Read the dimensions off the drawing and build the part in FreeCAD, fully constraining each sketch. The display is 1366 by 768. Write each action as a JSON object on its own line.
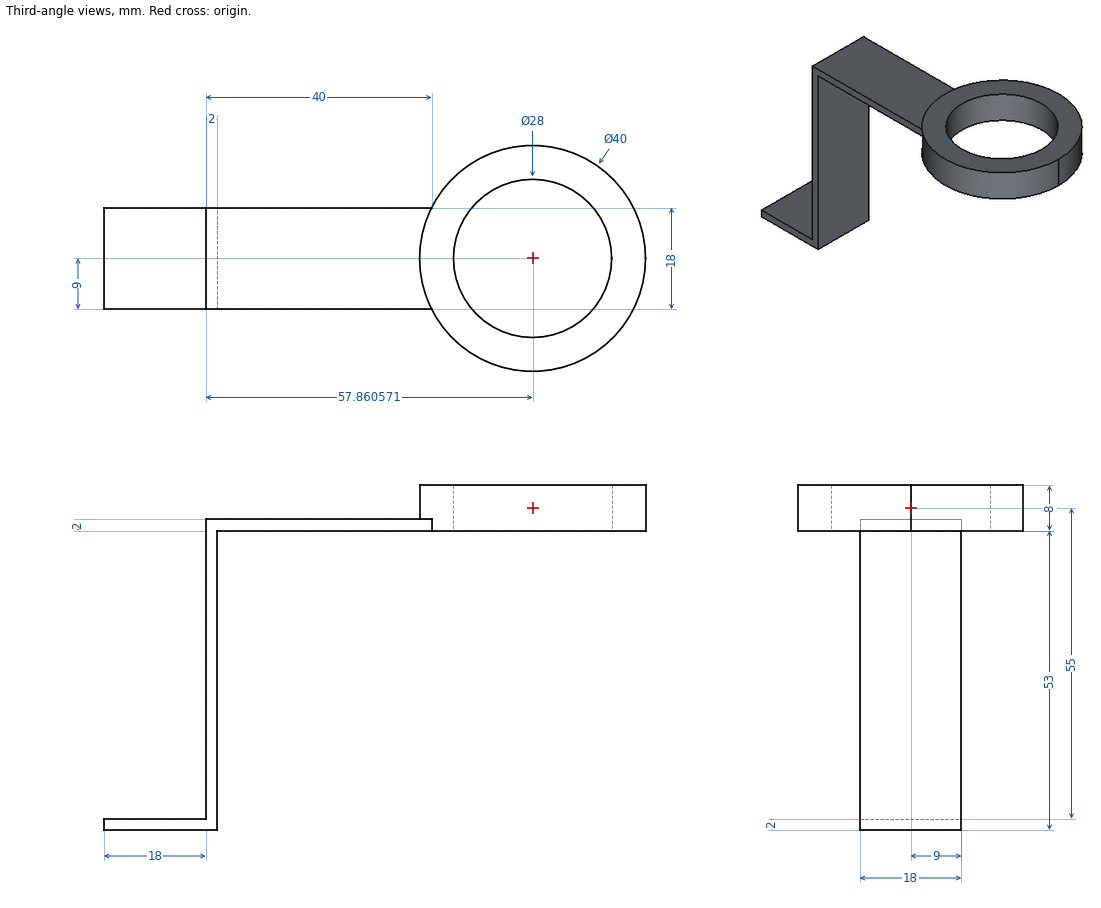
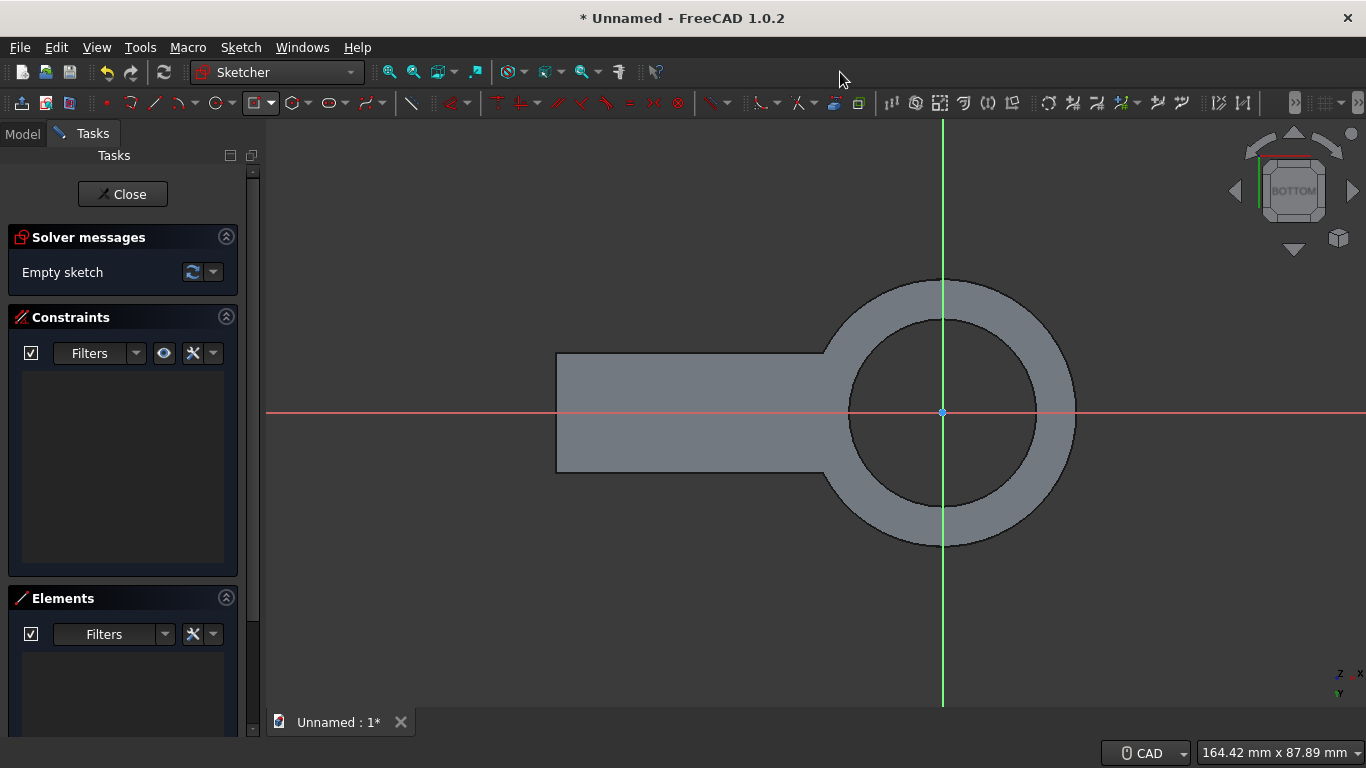
{"action": "scroll", "coordinate": [482, 413], "scroll_direction": "up", "scroll_amount": 6}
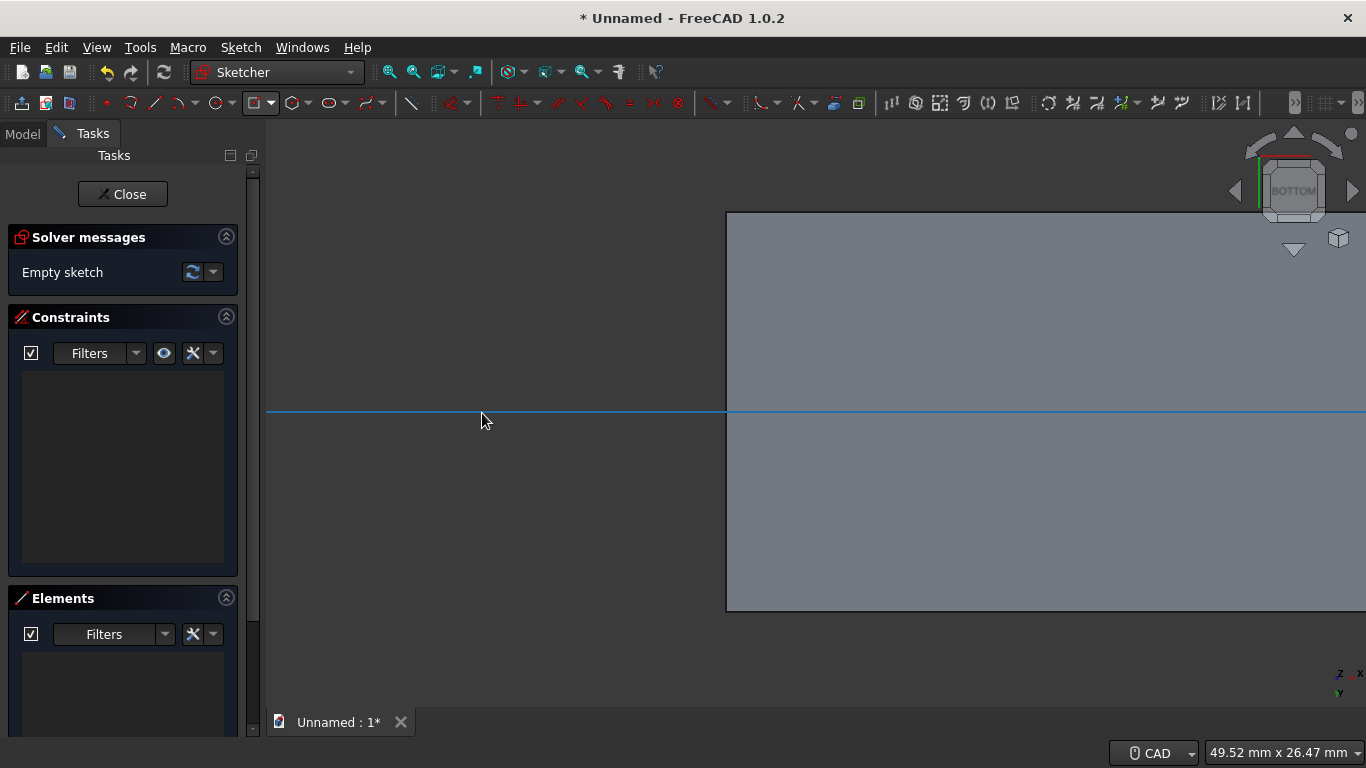
{"action": "left_click", "coordinate": [274, 104]}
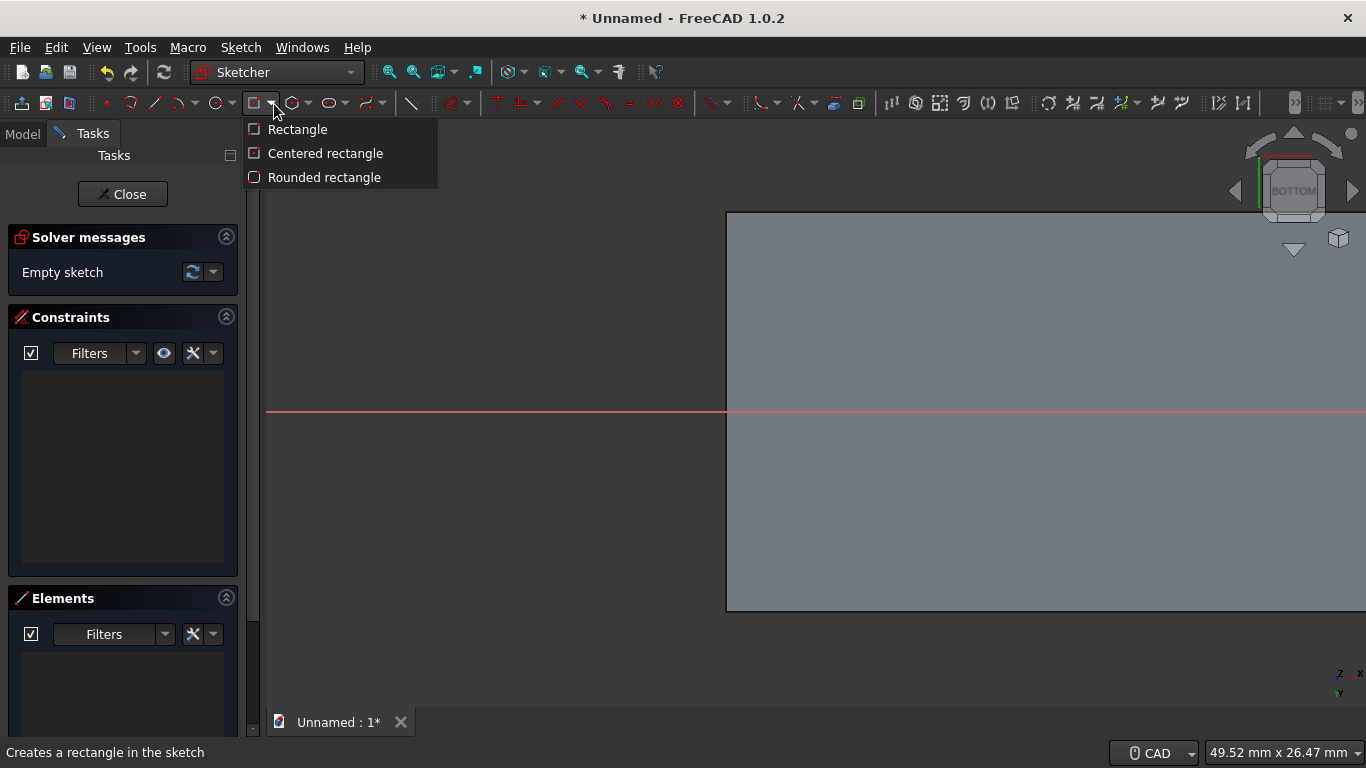
{"action": "left_click", "coordinate": [340, 129]}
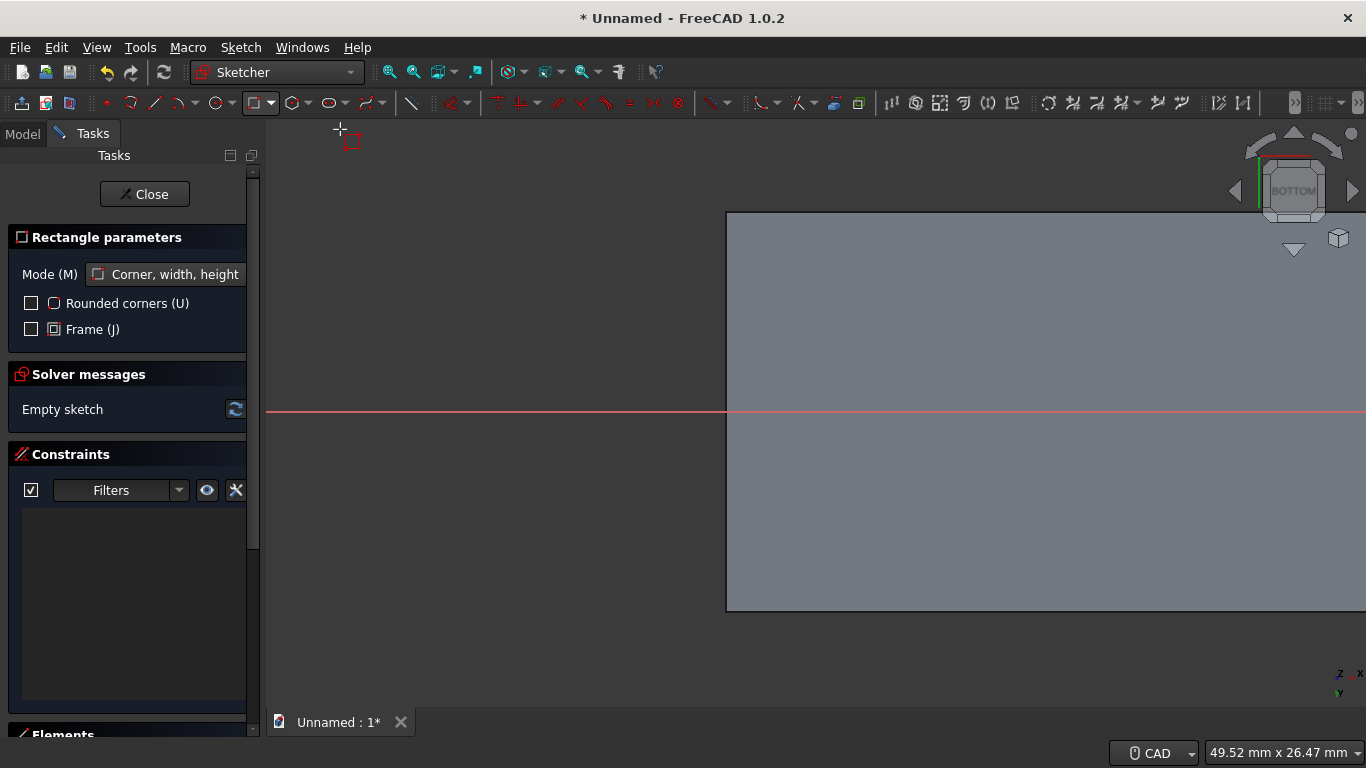
{"action": "left_click", "coordinate": [726, 212]}
{"action": "mouse_move", "coordinate": [770, 612]}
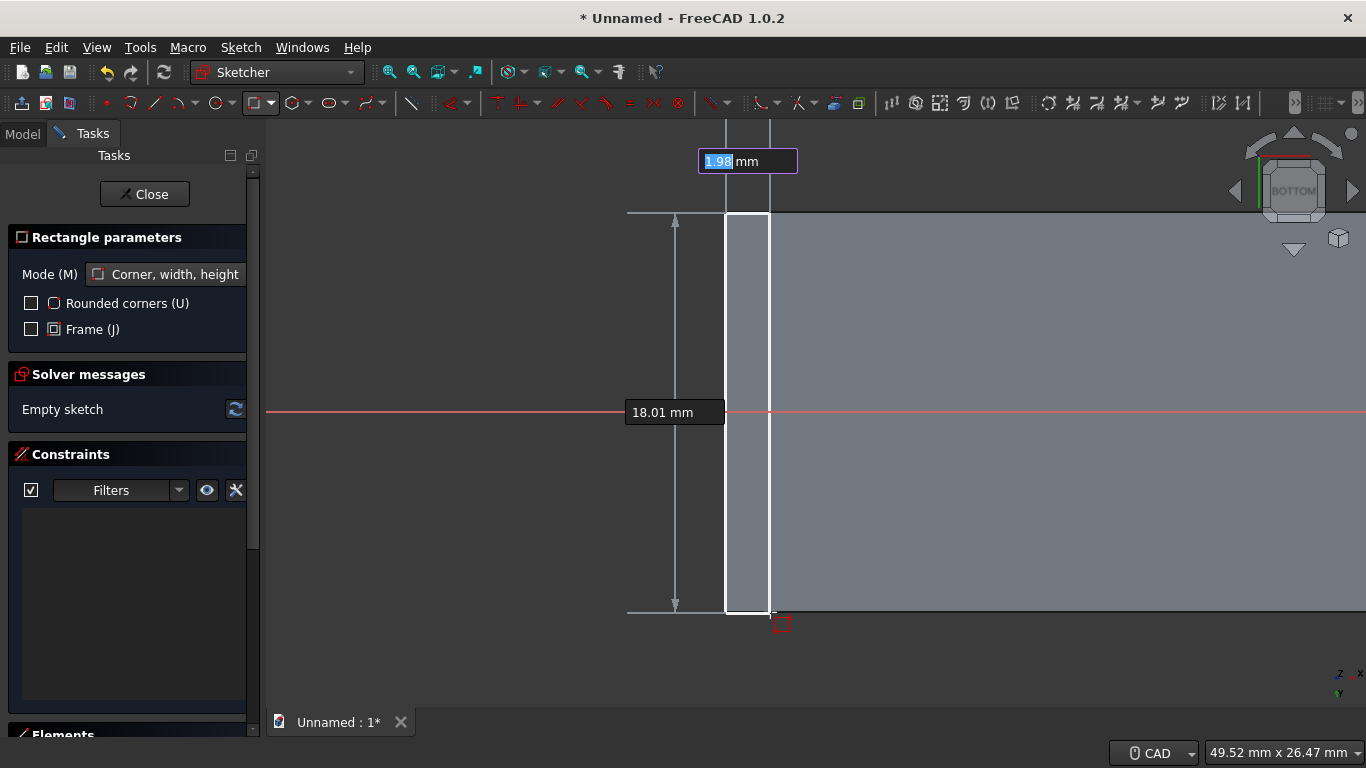
{"action": "type", "text": "2"}
{"action": "key", "text": "Tab"}
{"action": "type", "text": "18"}
{"action": "key", "text": "Return"}
{"action": "key", "text": "Escape"}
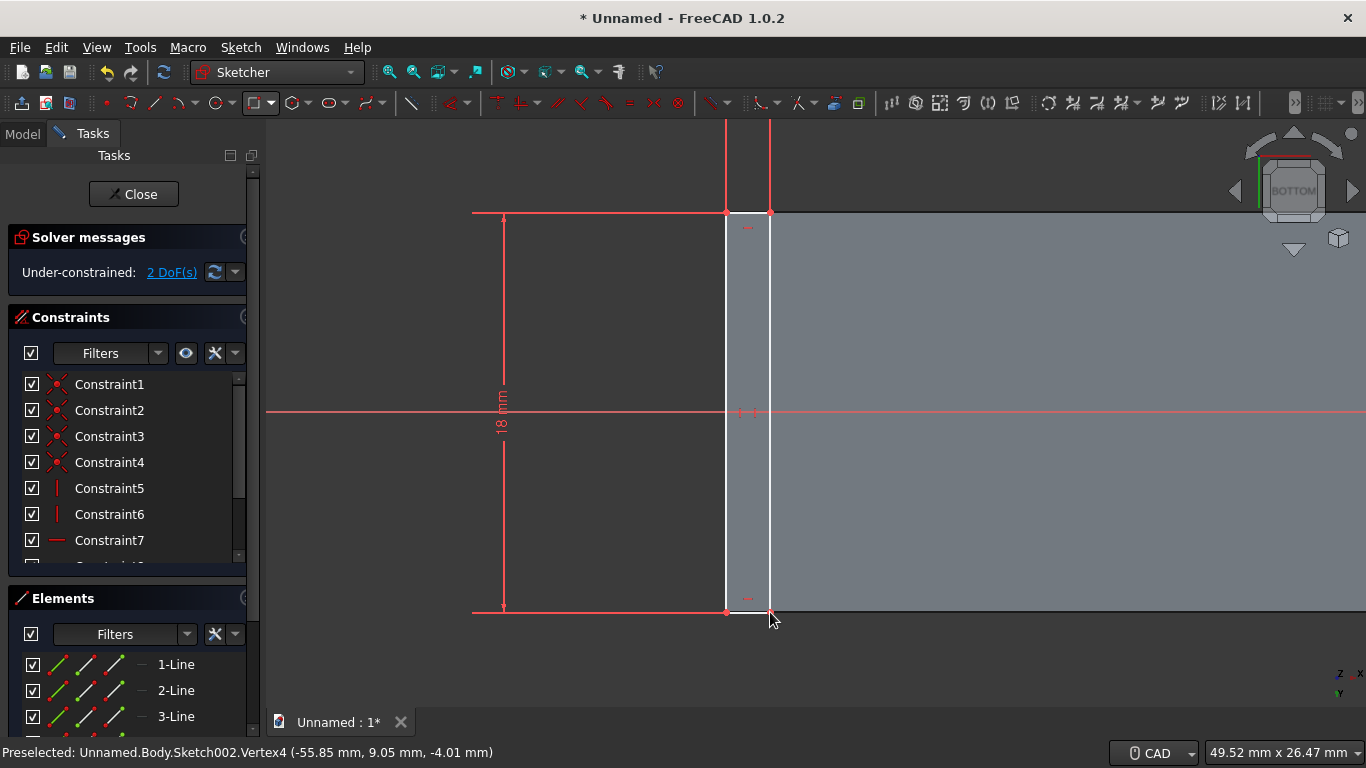
{"action": "left_click", "coordinate": [450, 104]}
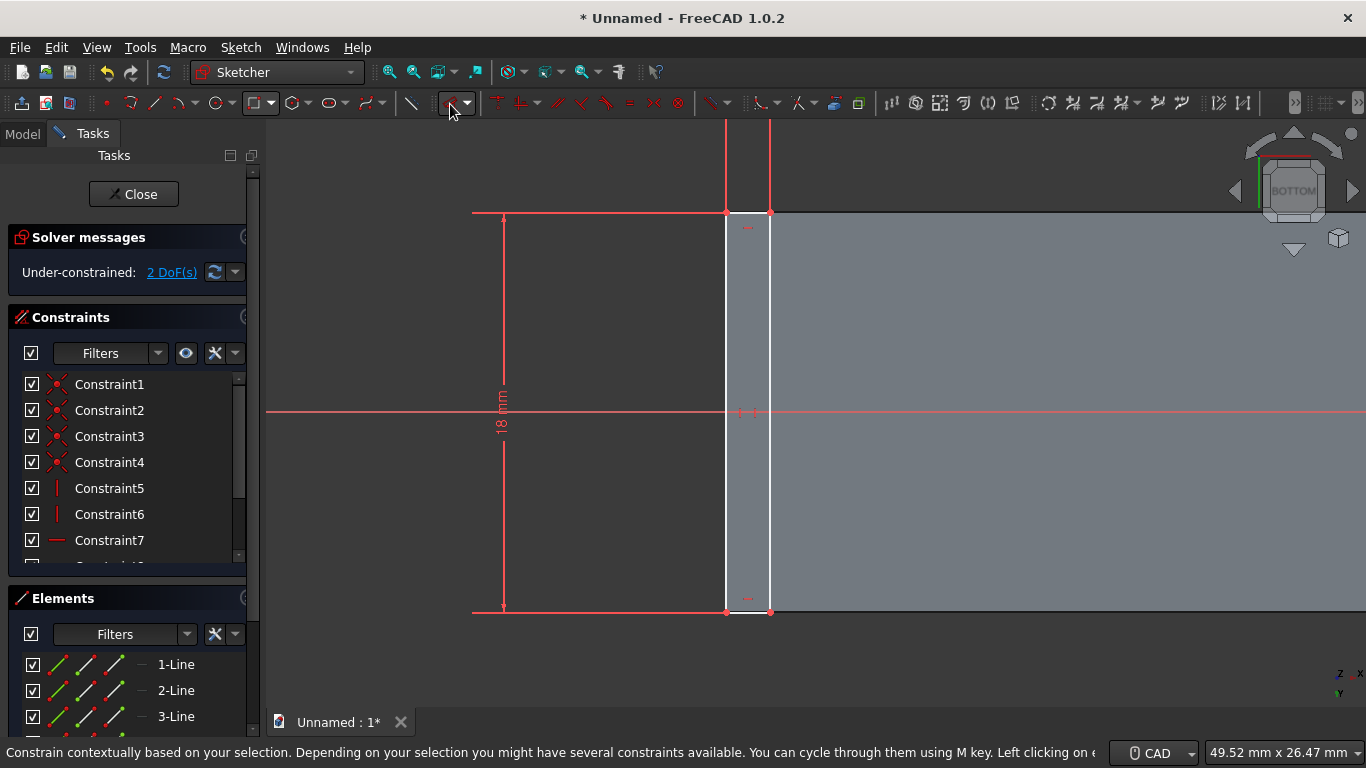
{"action": "left_click", "coordinate": [726, 213]}
{"action": "left_click", "coordinate": [692, 312]}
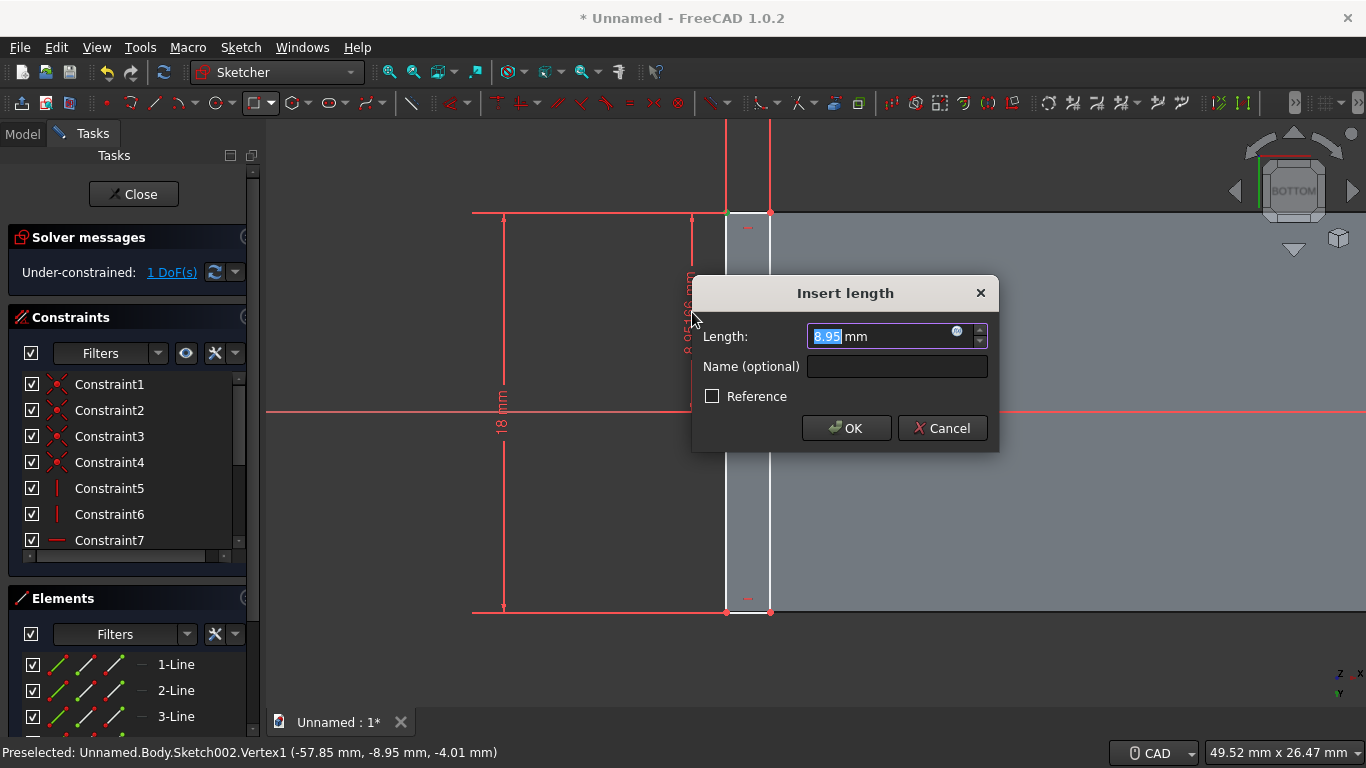
{"action": "type", "text": "9"}
{"action": "key", "text": "Return"}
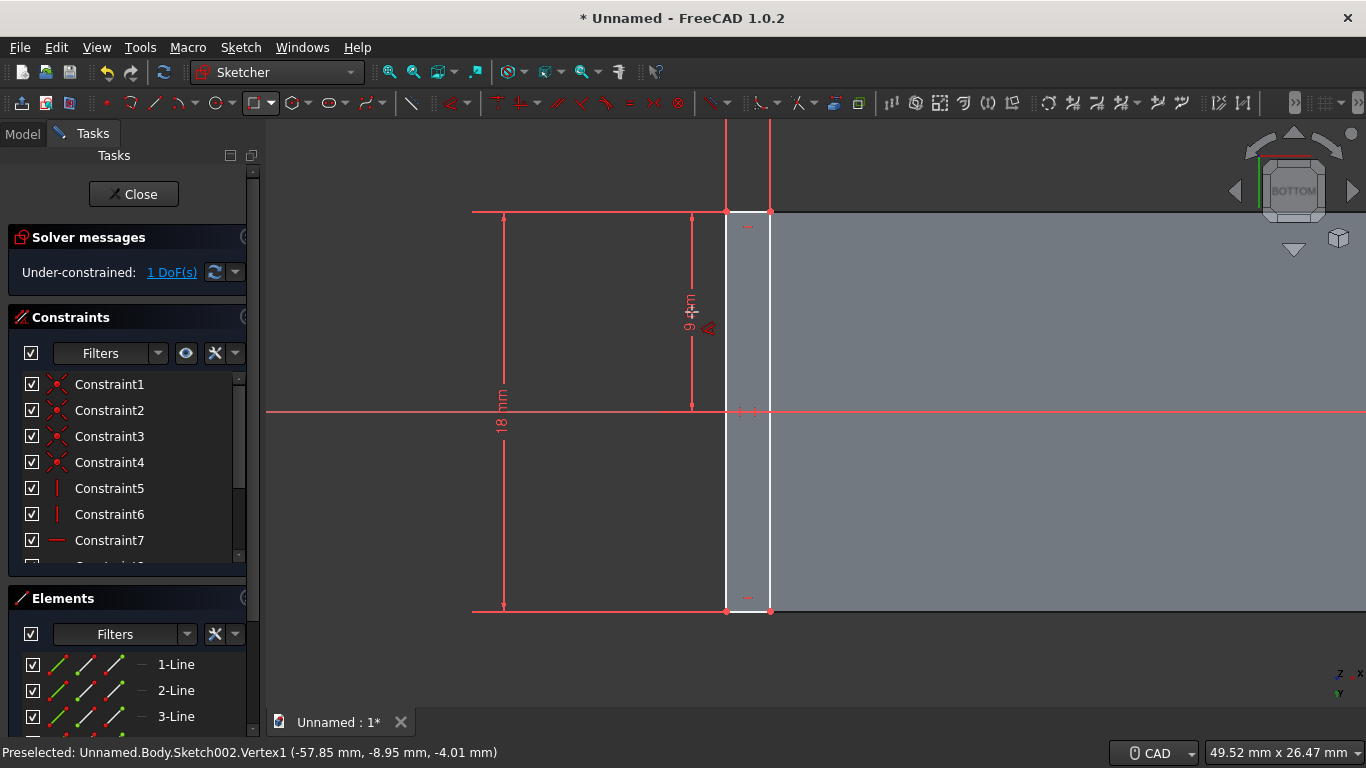
{"action": "left_click", "coordinate": [726, 212]}
{"action": "left_click", "coordinate": [963, 178]}